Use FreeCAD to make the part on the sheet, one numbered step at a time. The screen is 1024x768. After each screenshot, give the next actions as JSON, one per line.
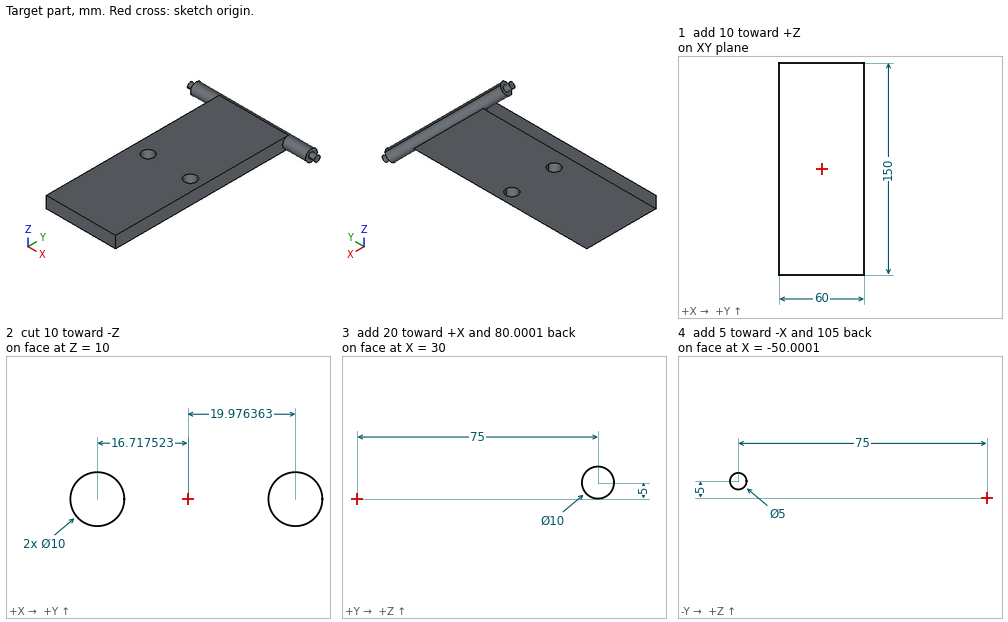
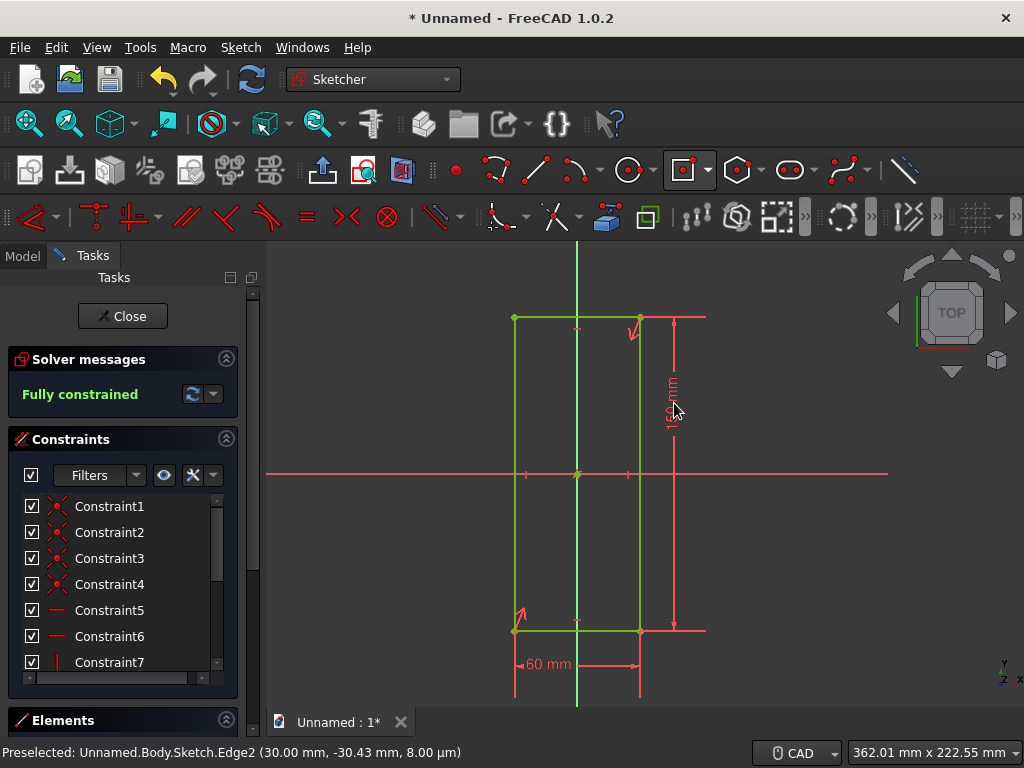
{"action": "left_click", "coordinate": [123, 316]}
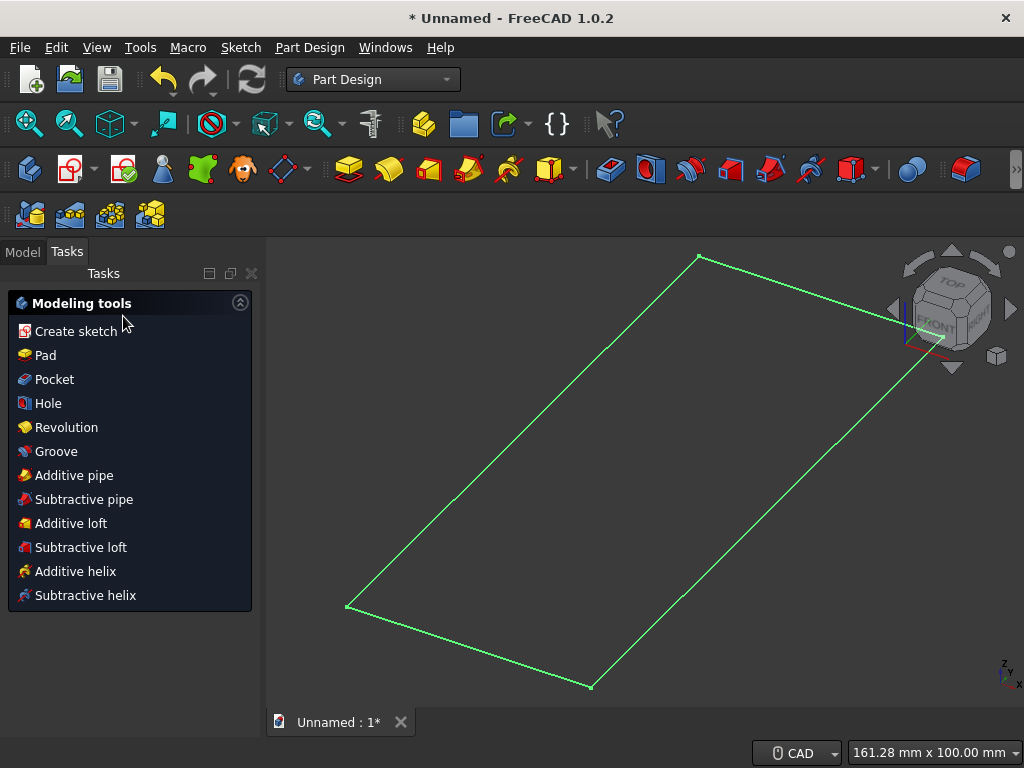
{"action": "left_click", "coordinate": [350, 170]}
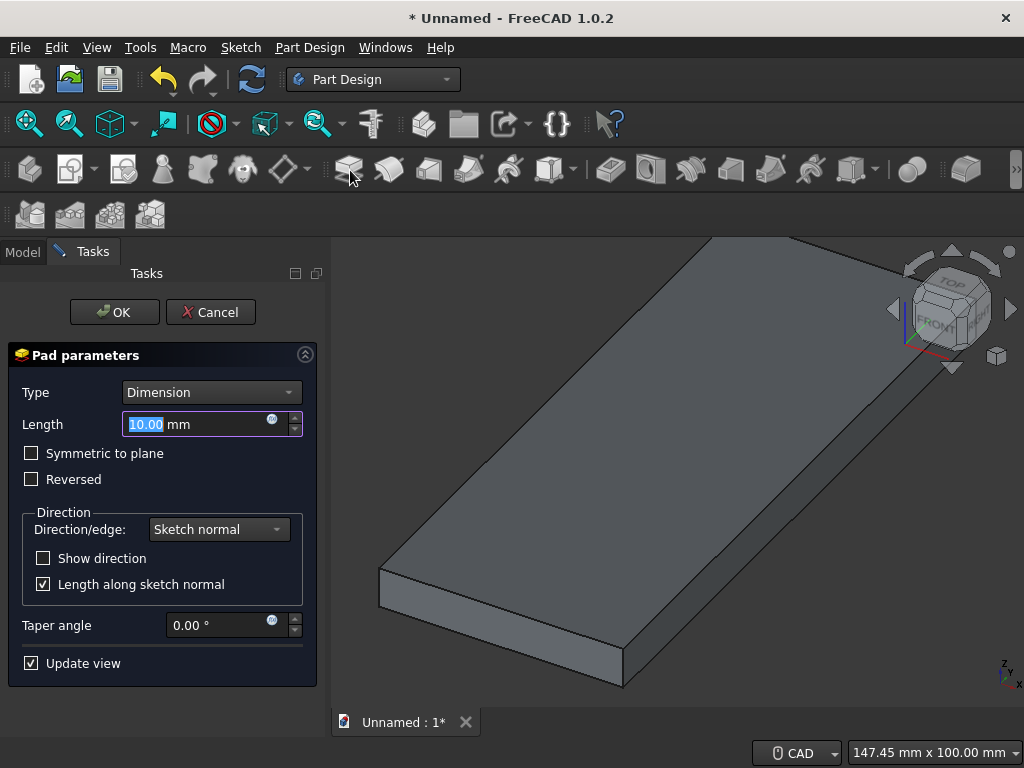
{"action": "type", "text": "10"}
{"action": "key", "text": "Tab"}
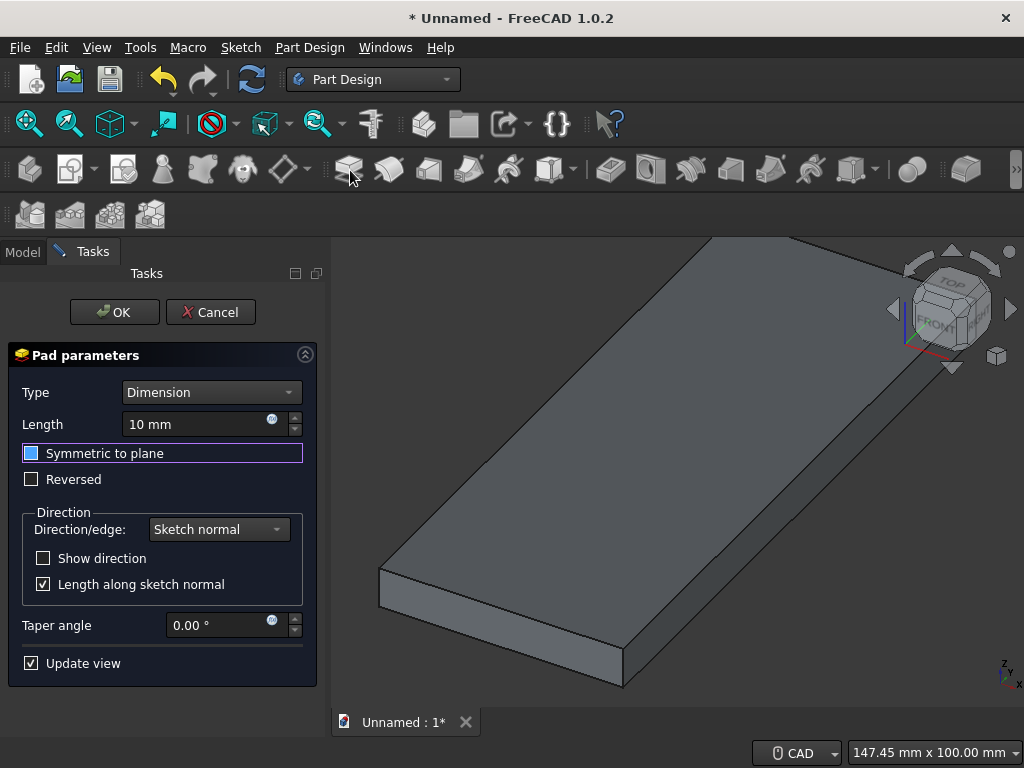
{"action": "left_click", "coordinate": [115, 312]}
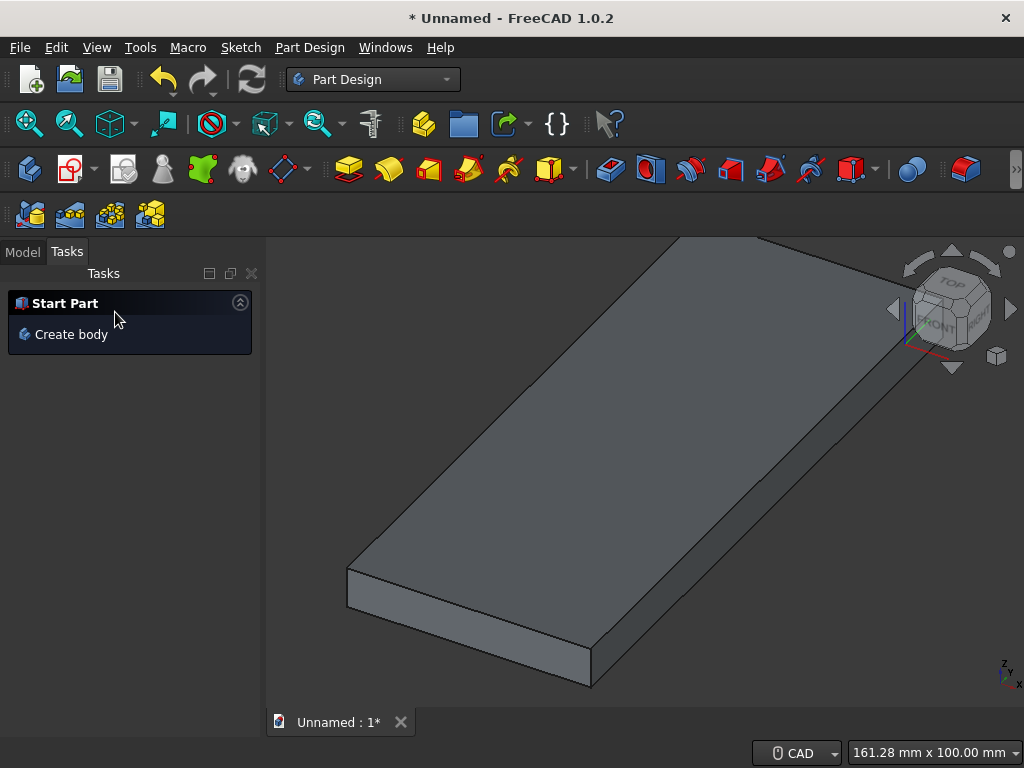
{"action": "left_click", "coordinate": [30, 124]}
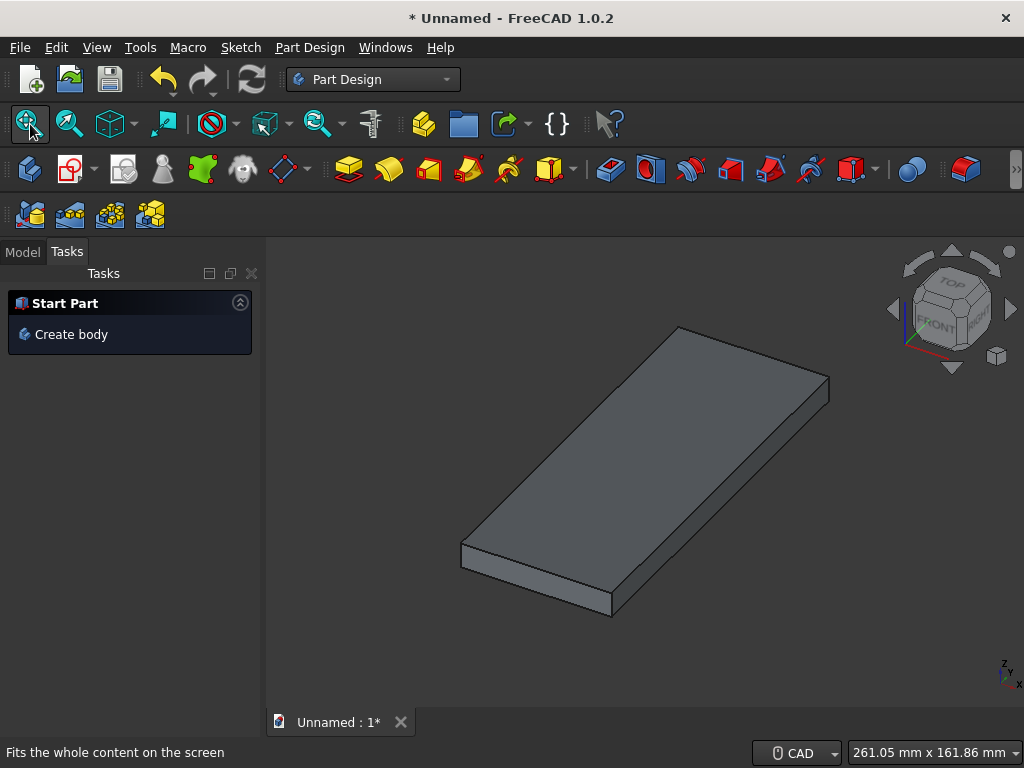
{"action": "left_click", "coordinate": [707, 397]}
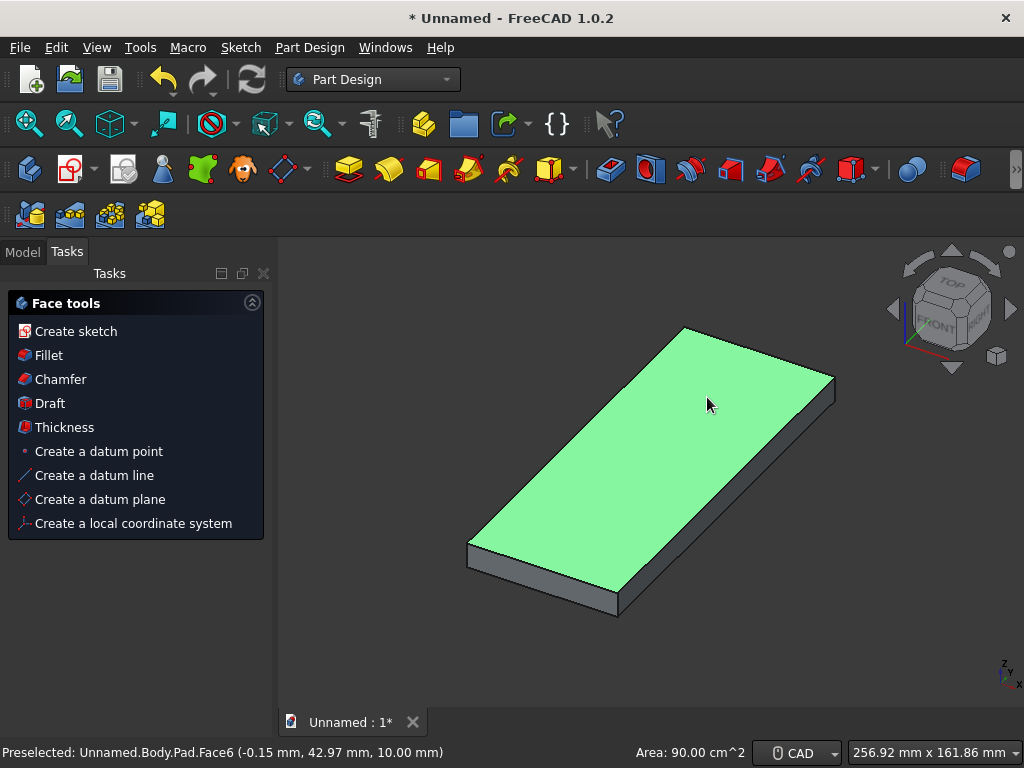
{"action": "left_click", "coordinate": [70, 170]}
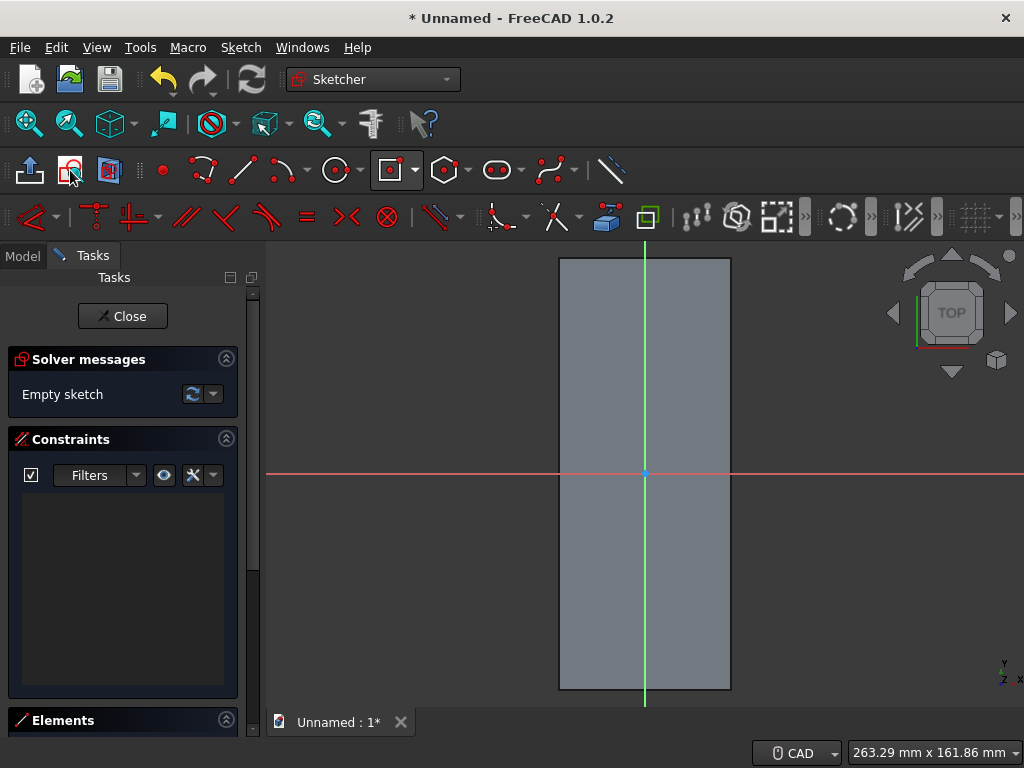
{"action": "scroll", "coordinate": [692, 474], "scroll_direction": "up", "scroll_amount": 5}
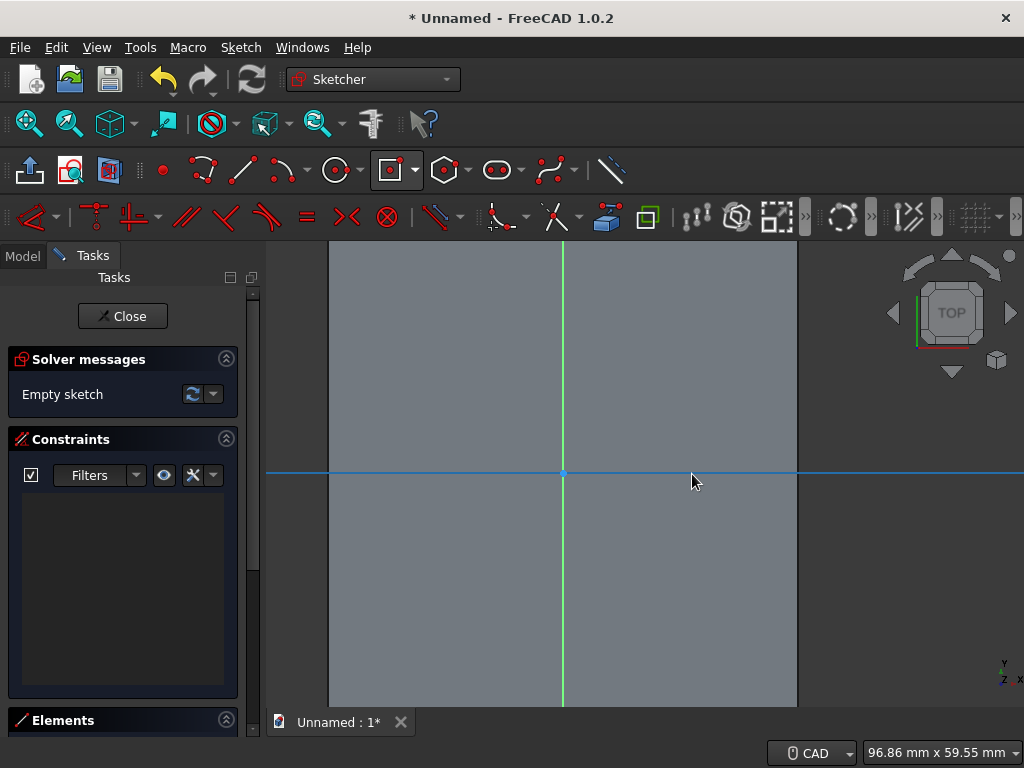
{"action": "left_click", "coordinate": [336, 170]}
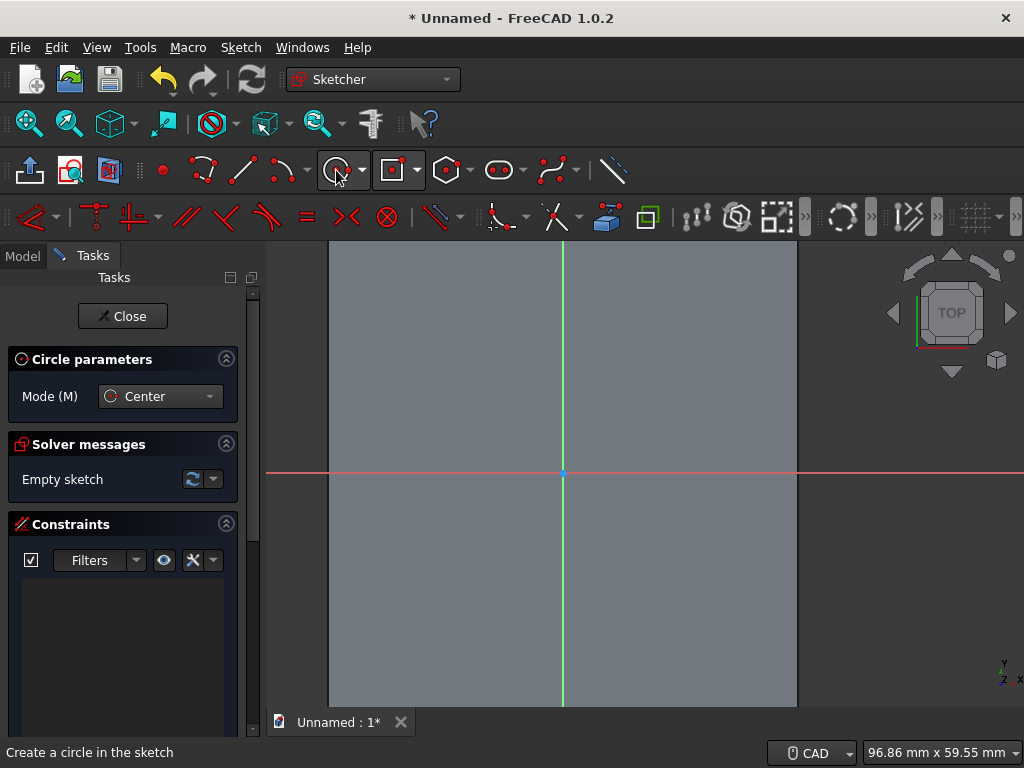
{"action": "left_click", "coordinate": [432, 473]}
{"action": "left_click", "coordinate": [460, 445]}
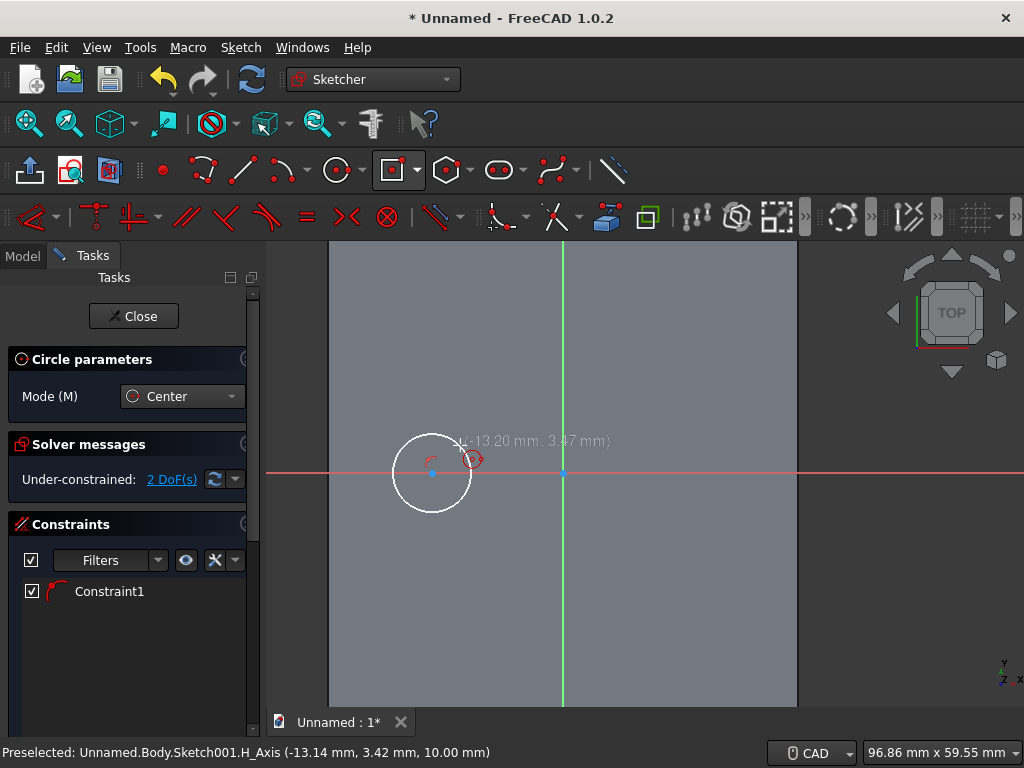
{"action": "left_click", "coordinate": [720, 473]}
{"action": "left_click", "coordinate": [747, 445]}
{"action": "key", "text": "Escape"}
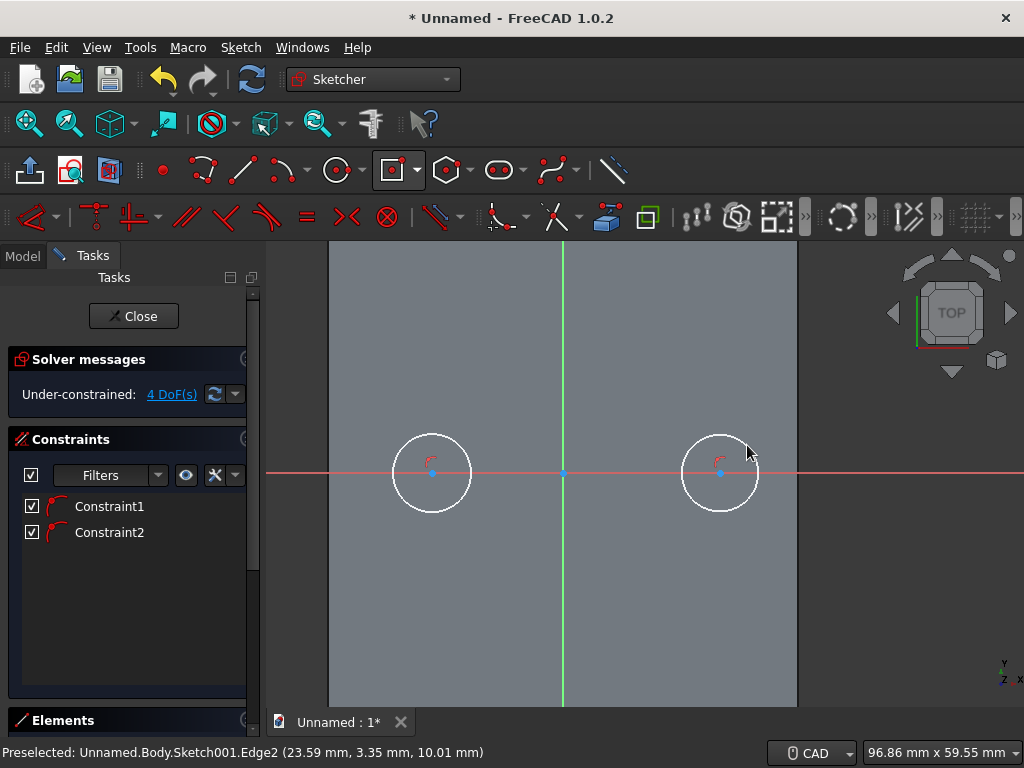
{"action": "left_click", "coordinate": [459, 445]}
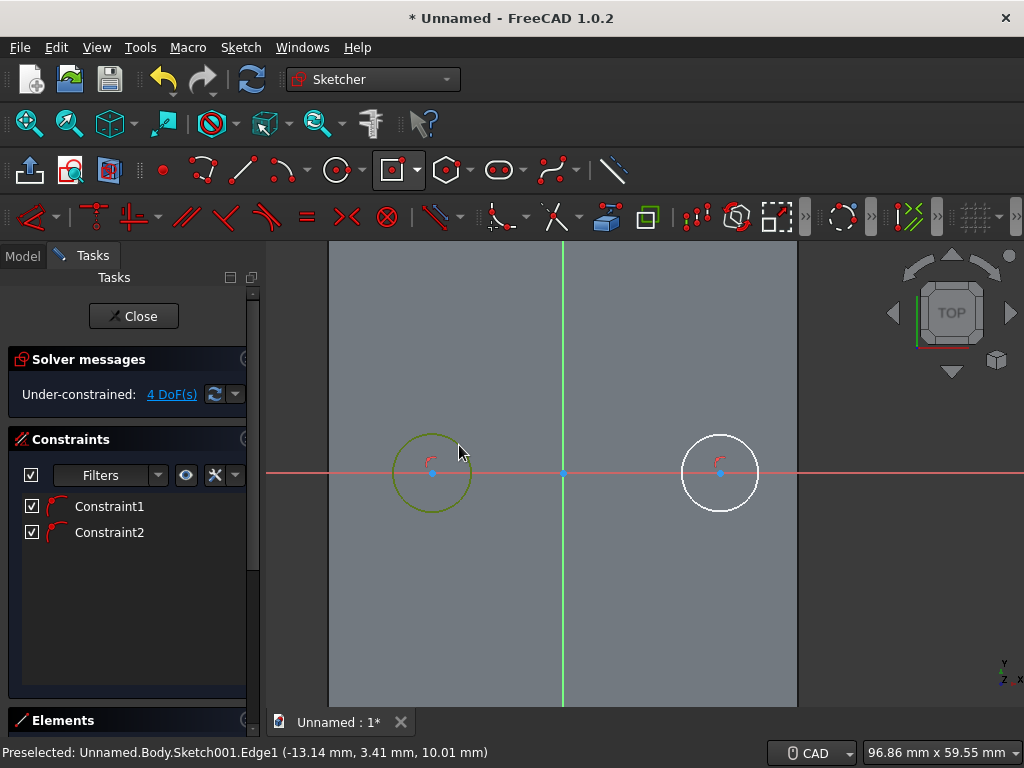
{"action": "left_click", "coordinate": [747, 446]}